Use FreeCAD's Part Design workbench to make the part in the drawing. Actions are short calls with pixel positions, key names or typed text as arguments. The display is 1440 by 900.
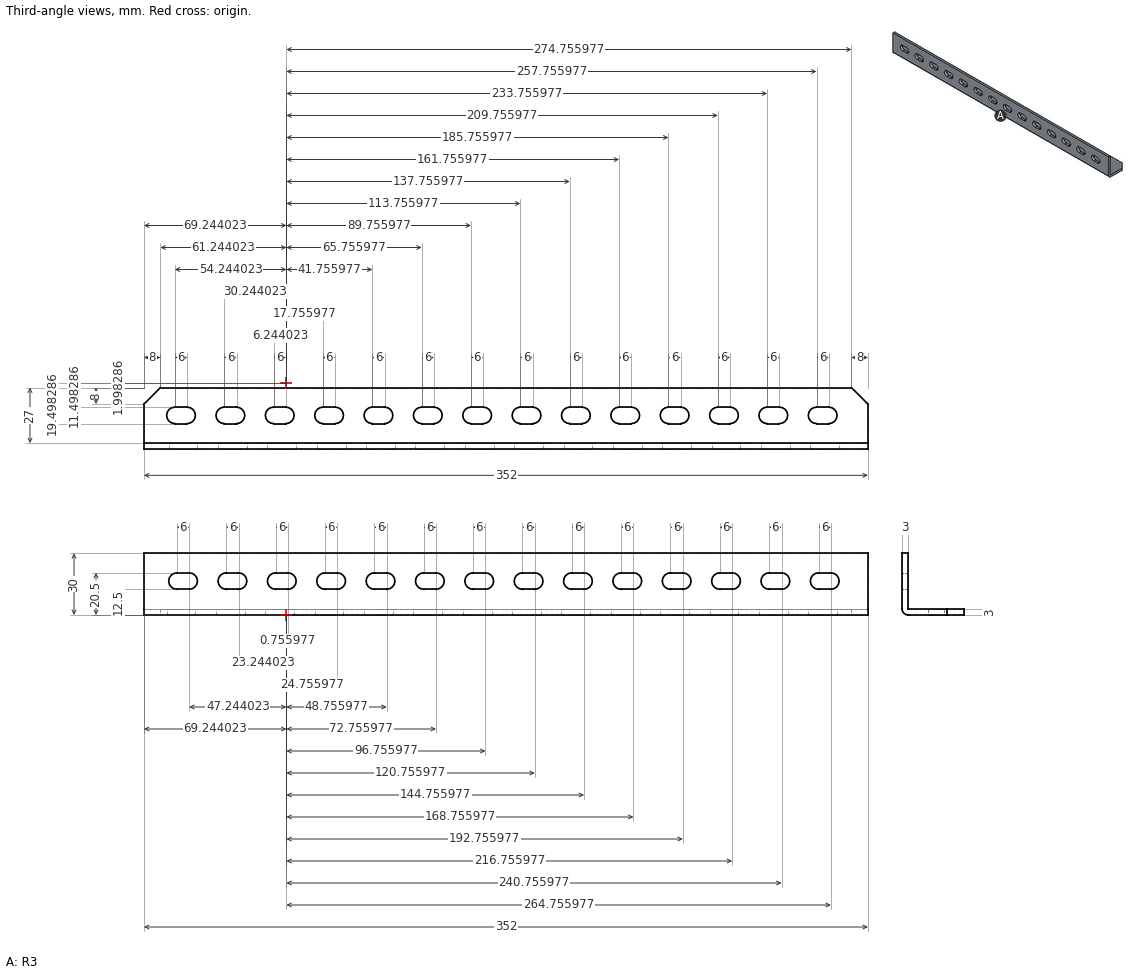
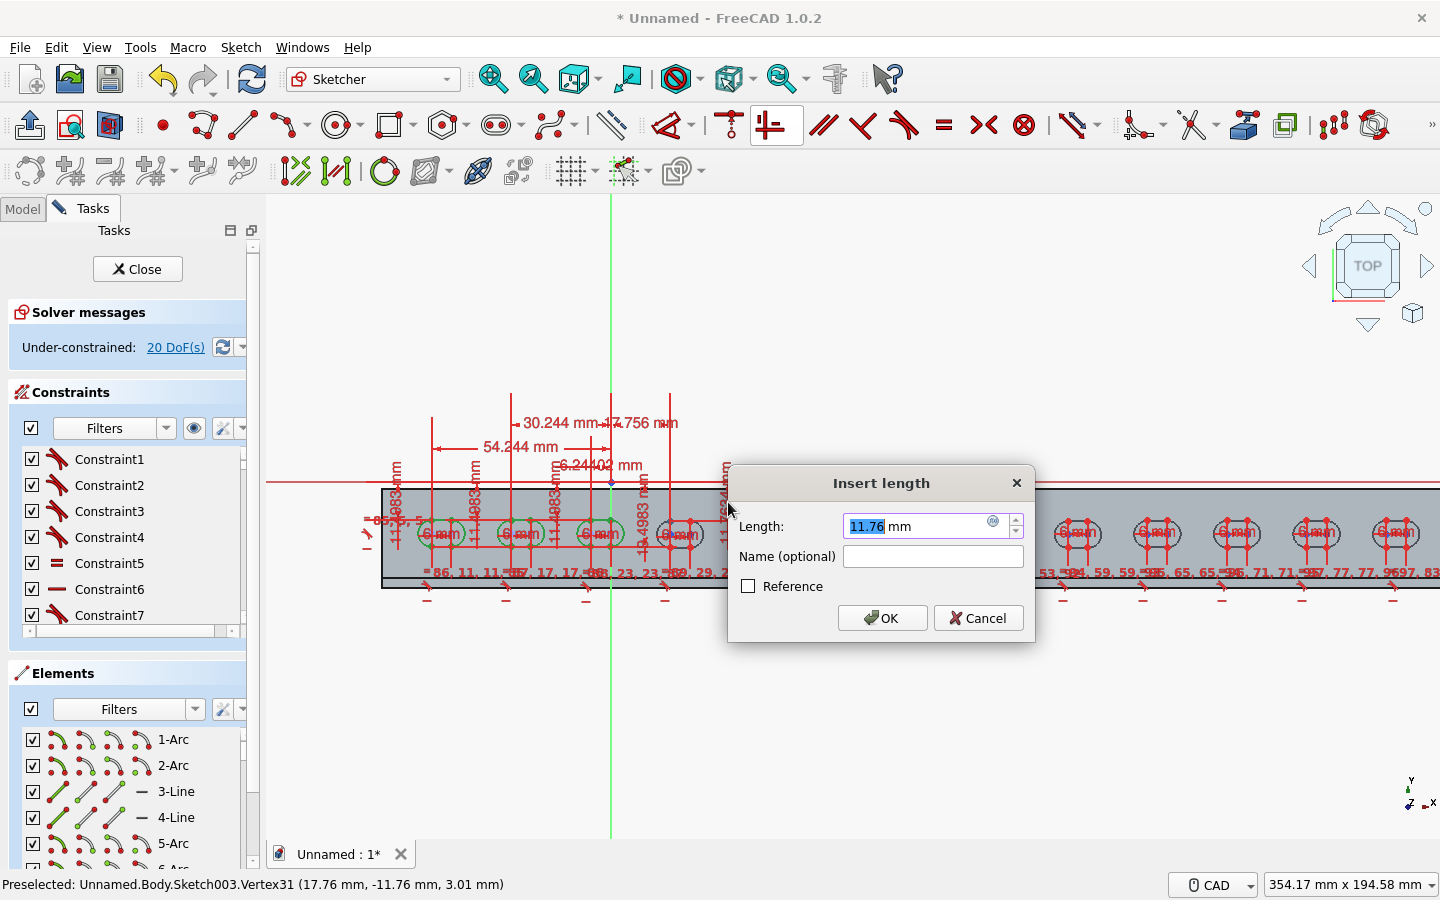
text(11.498286)
key(Return)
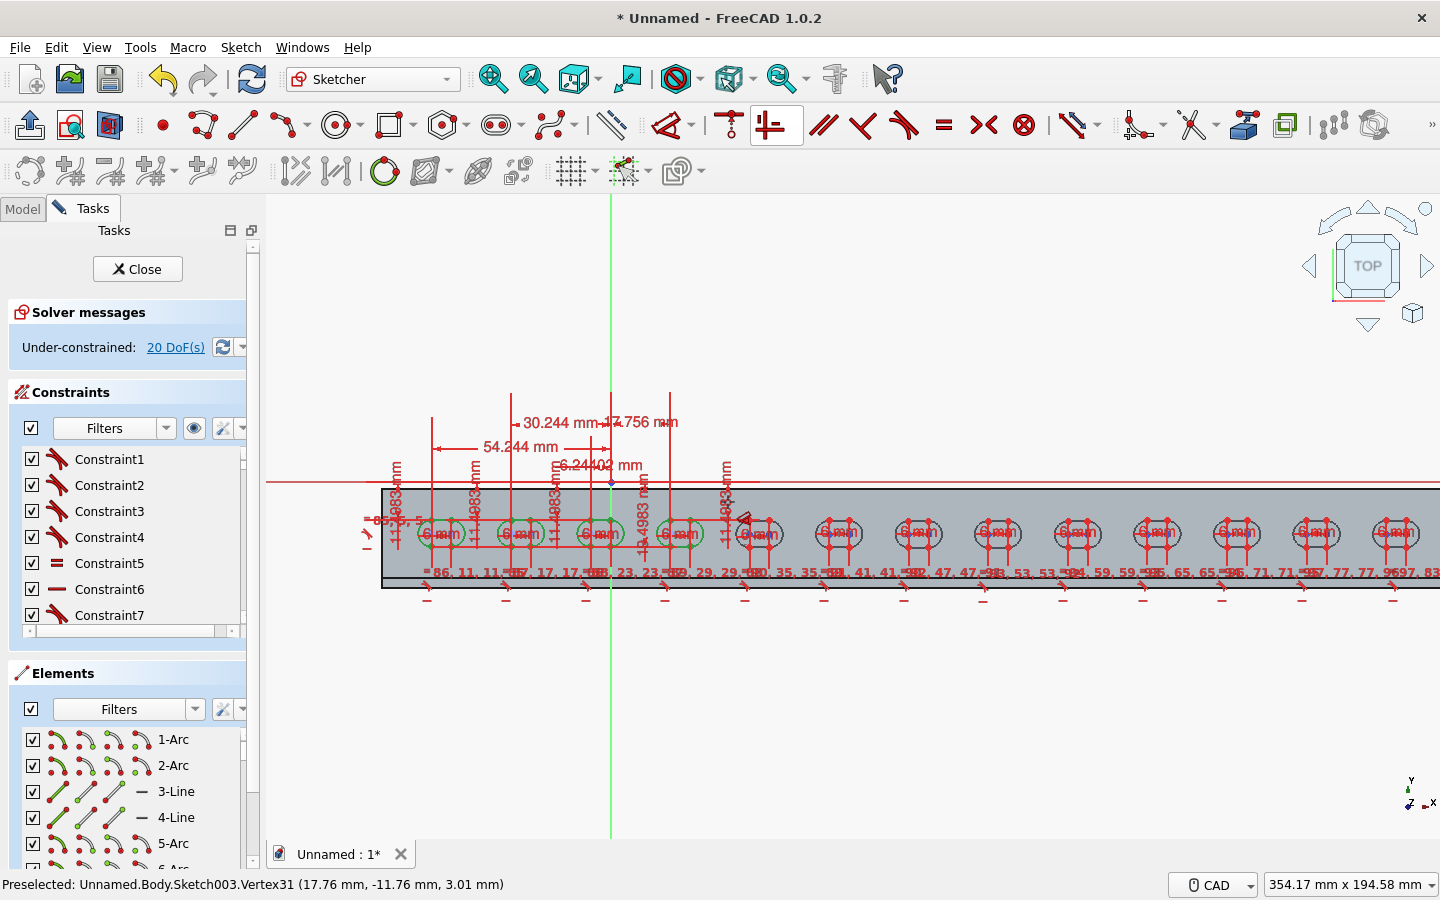
click(750, 521)
click(680, 448)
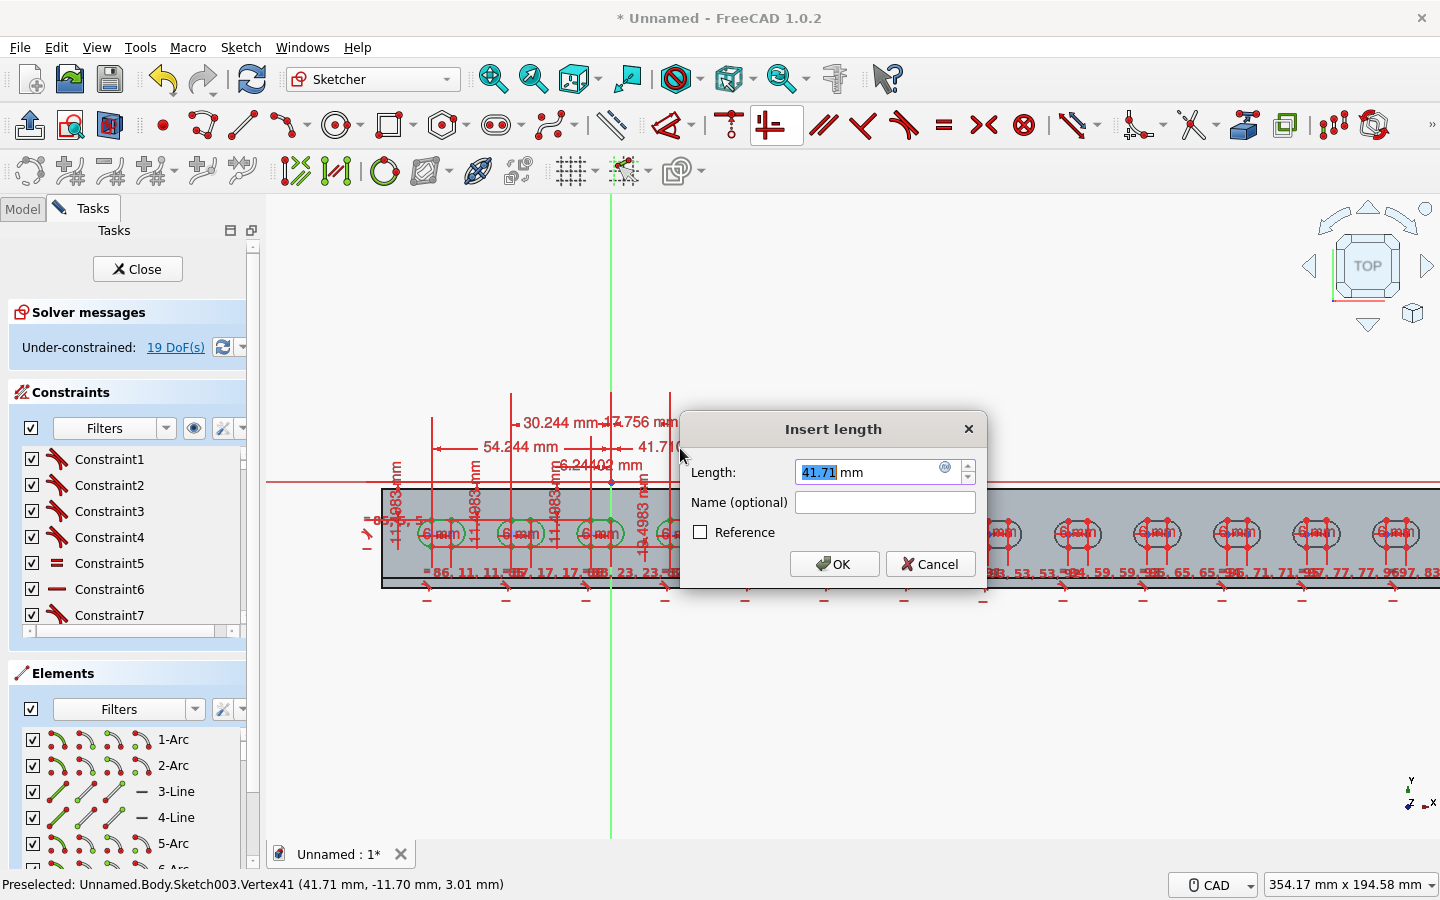
text(41.755977)
key(Return)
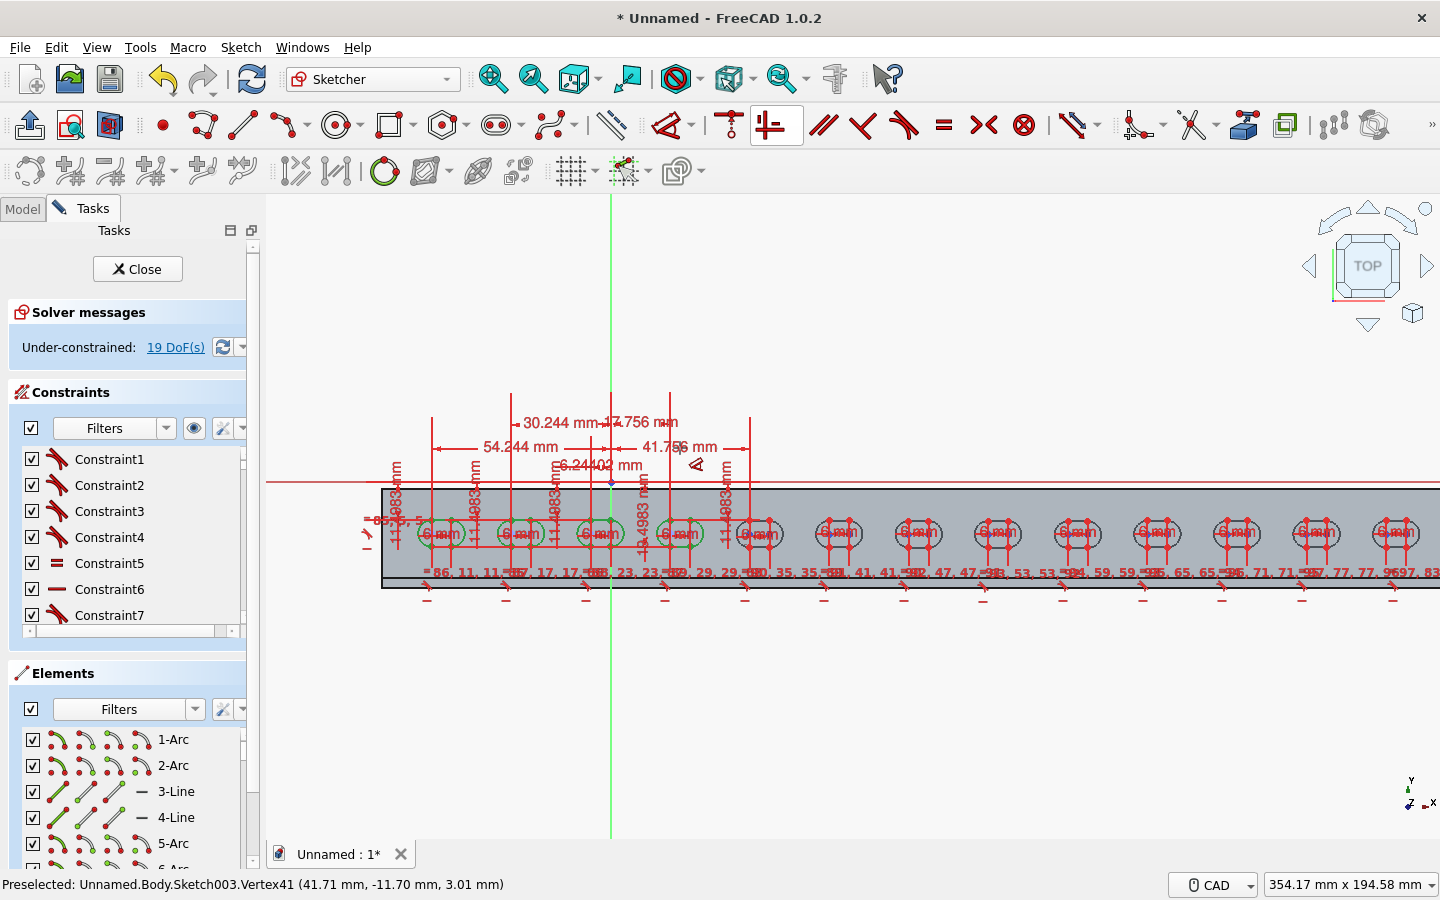
click(750, 521)
click(808, 502)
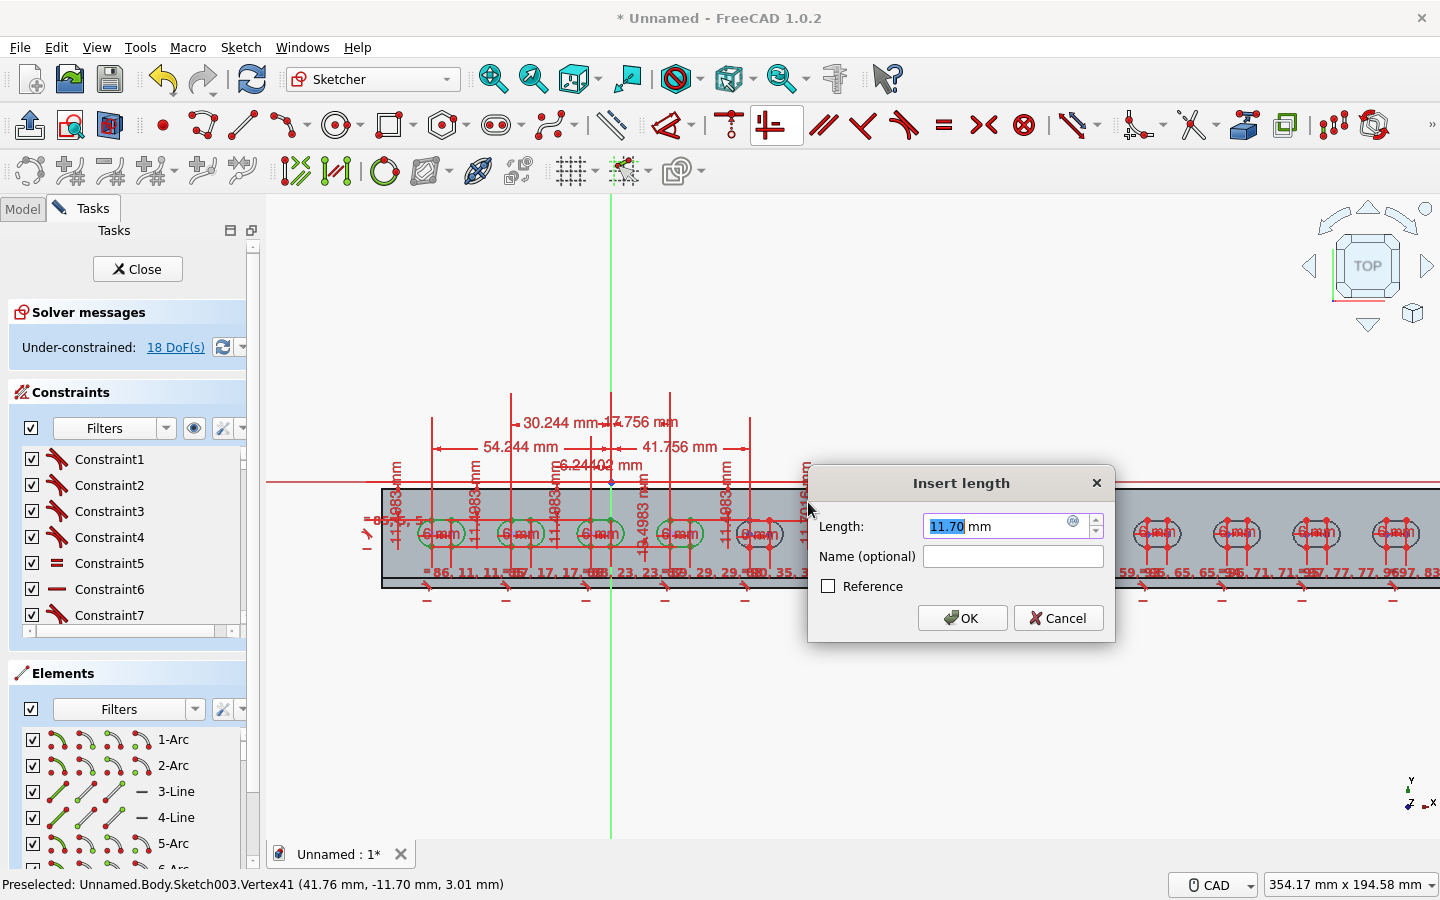
text(11.498286)
key(Return)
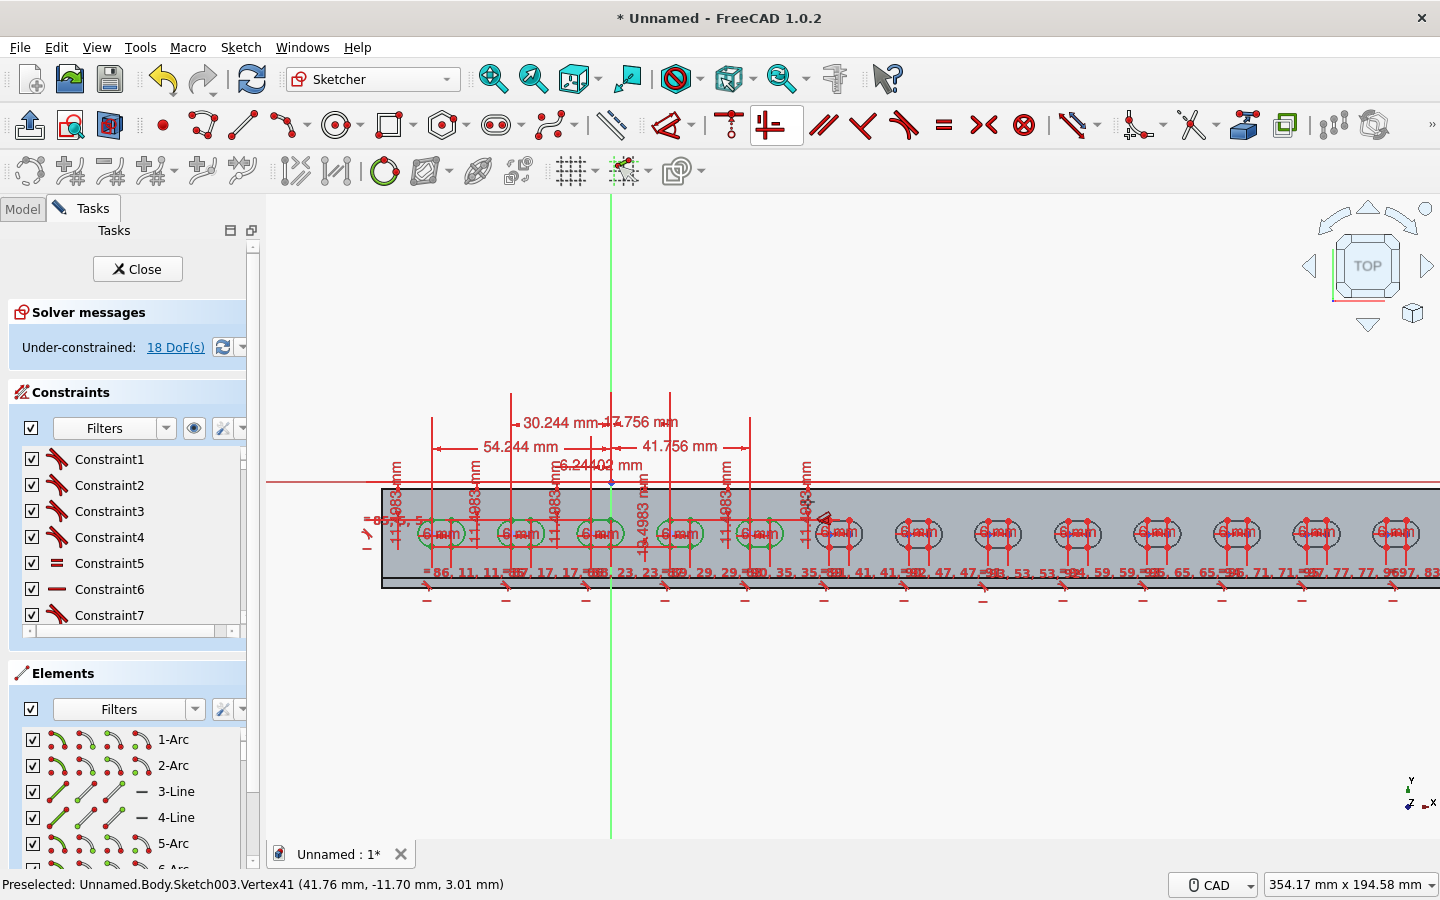
click(829, 521)
click(770, 448)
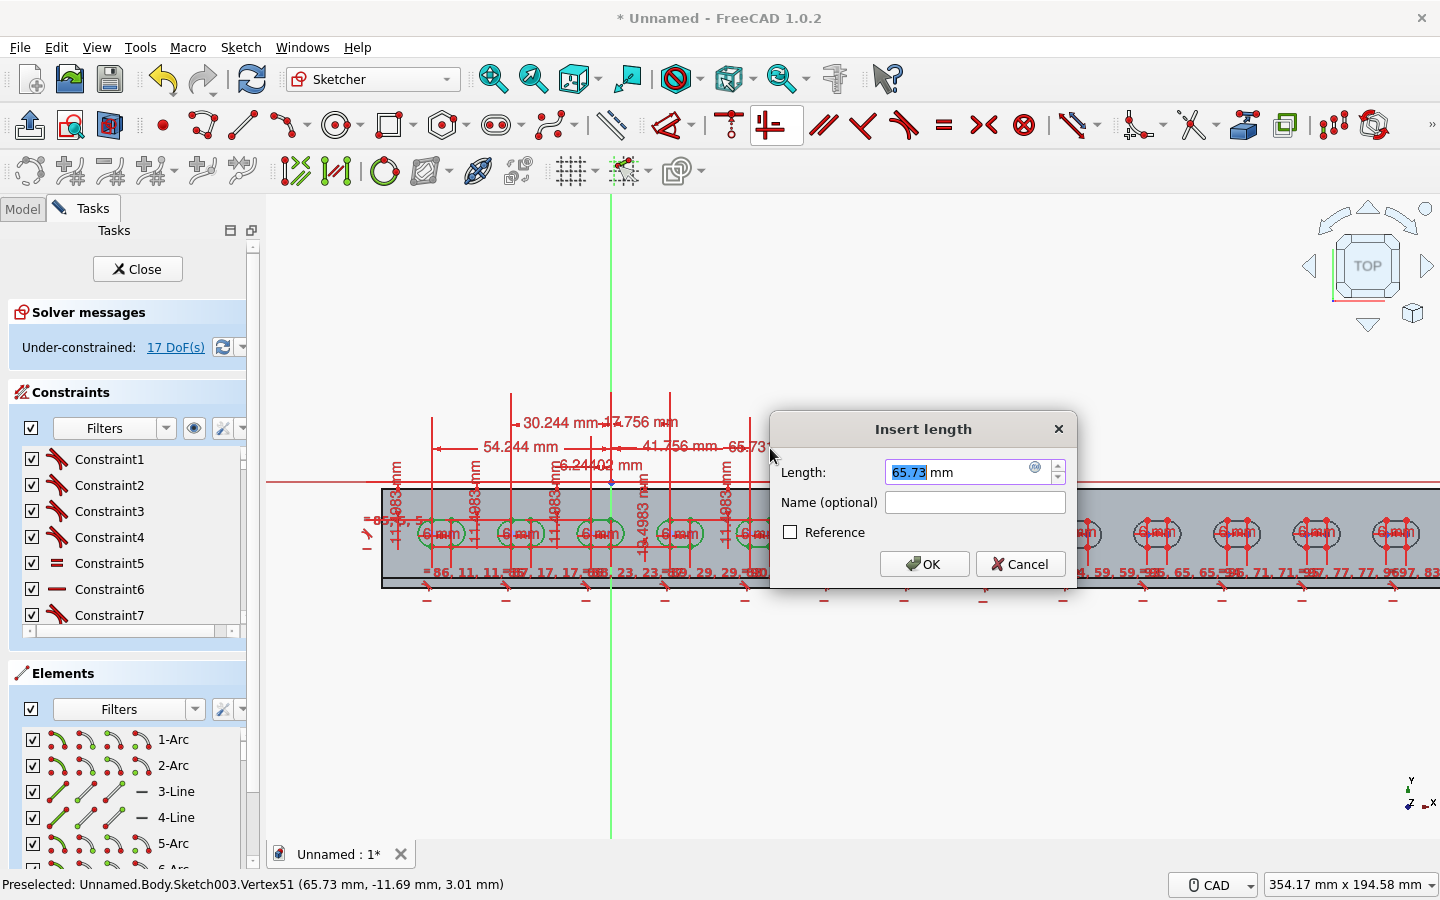
text(65.755977)
key(Return)